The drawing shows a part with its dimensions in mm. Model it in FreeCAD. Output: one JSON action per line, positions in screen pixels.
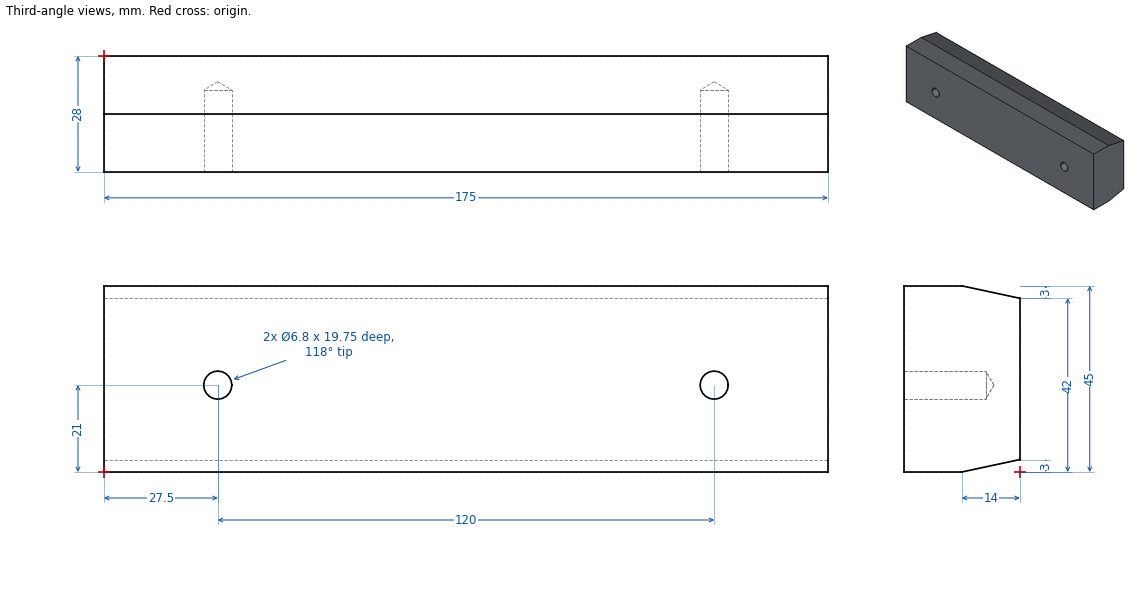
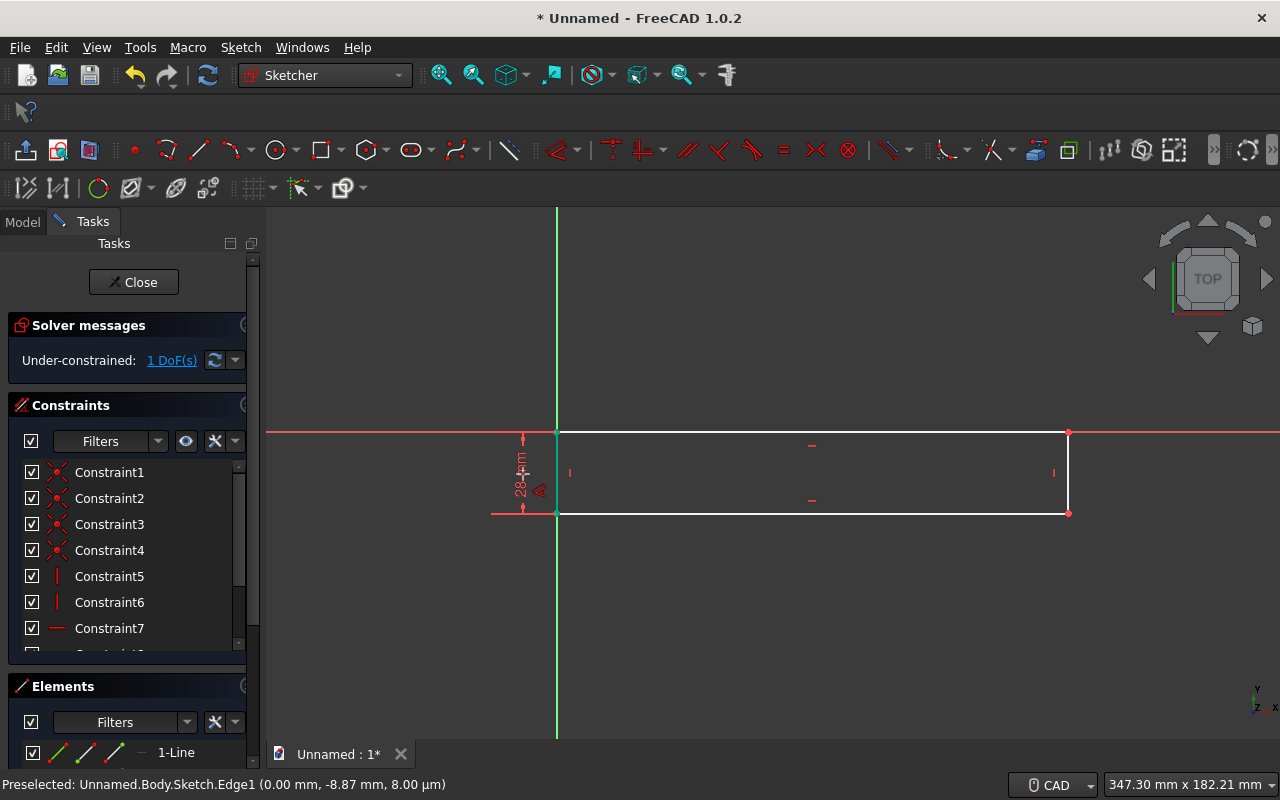
{"action": "left_click", "coordinate": [710, 514]}
{"action": "left_click", "coordinate": [812, 548]}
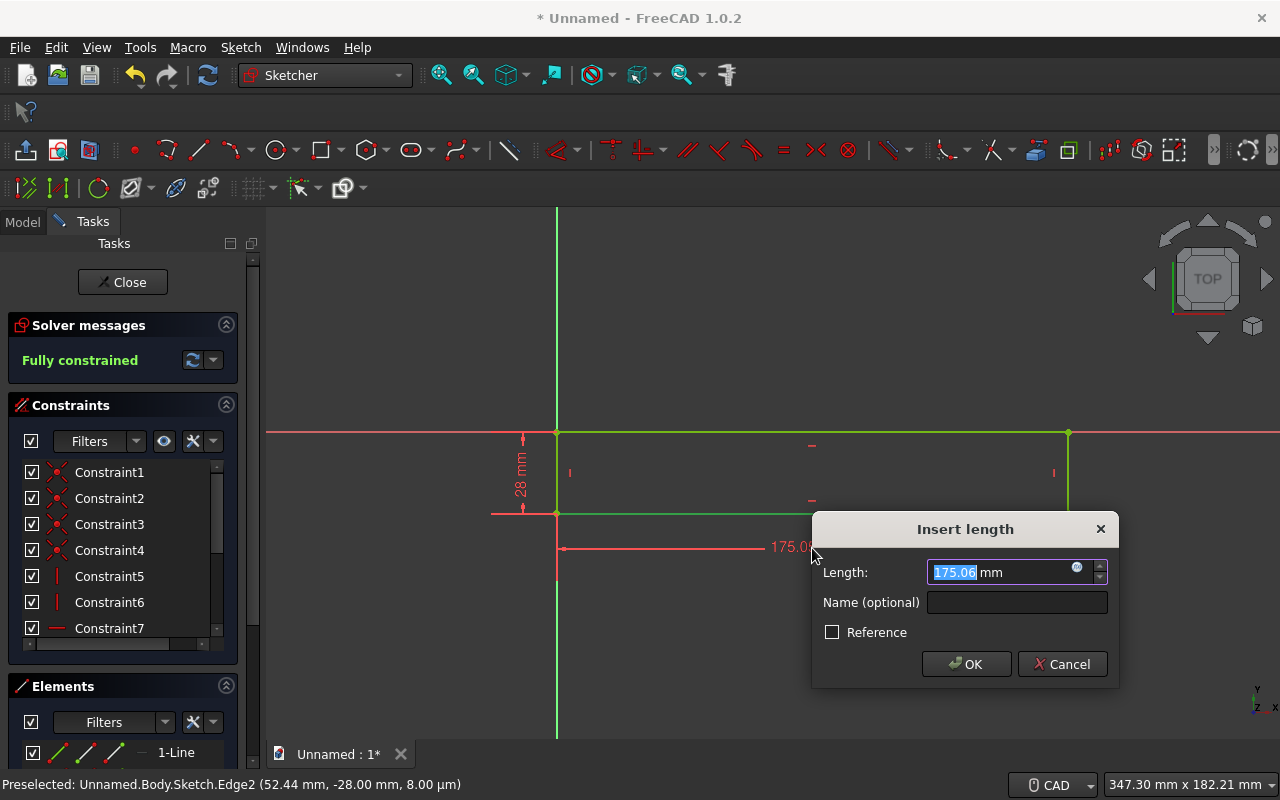
{"action": "type", "text": "175"}
{"action": "key", "text": "Return"}
{"action": "key", "text": "Escape"}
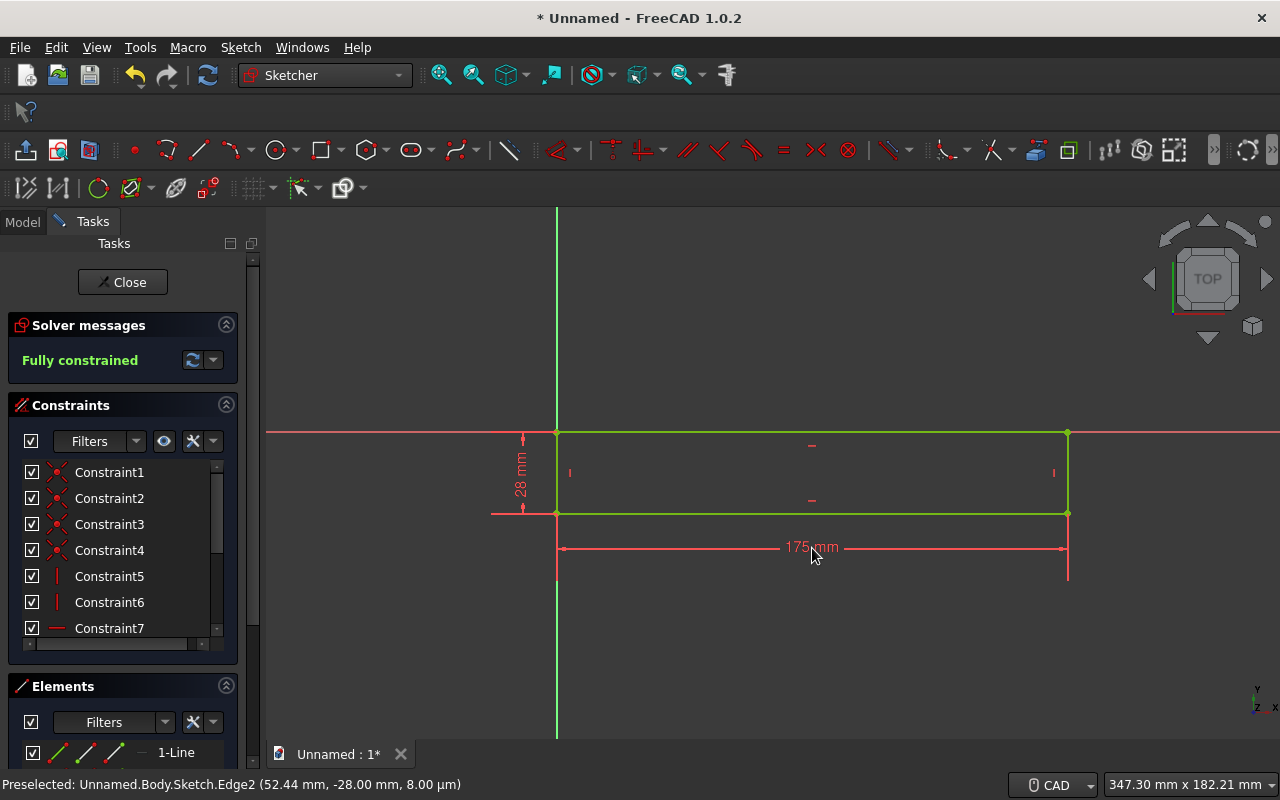
{"action": "left_click", "coordinate": [123, 282]}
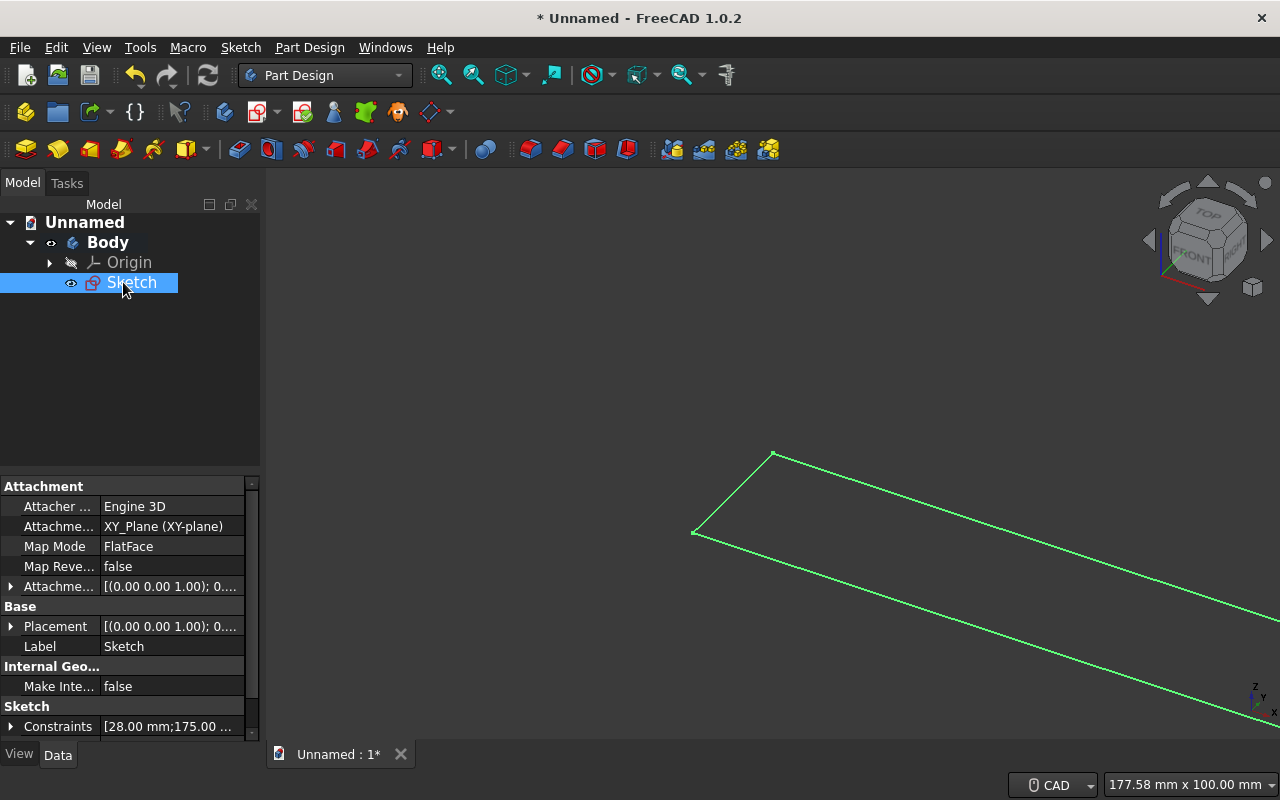
{"action": "left_click", "coordinate": [26, 150]}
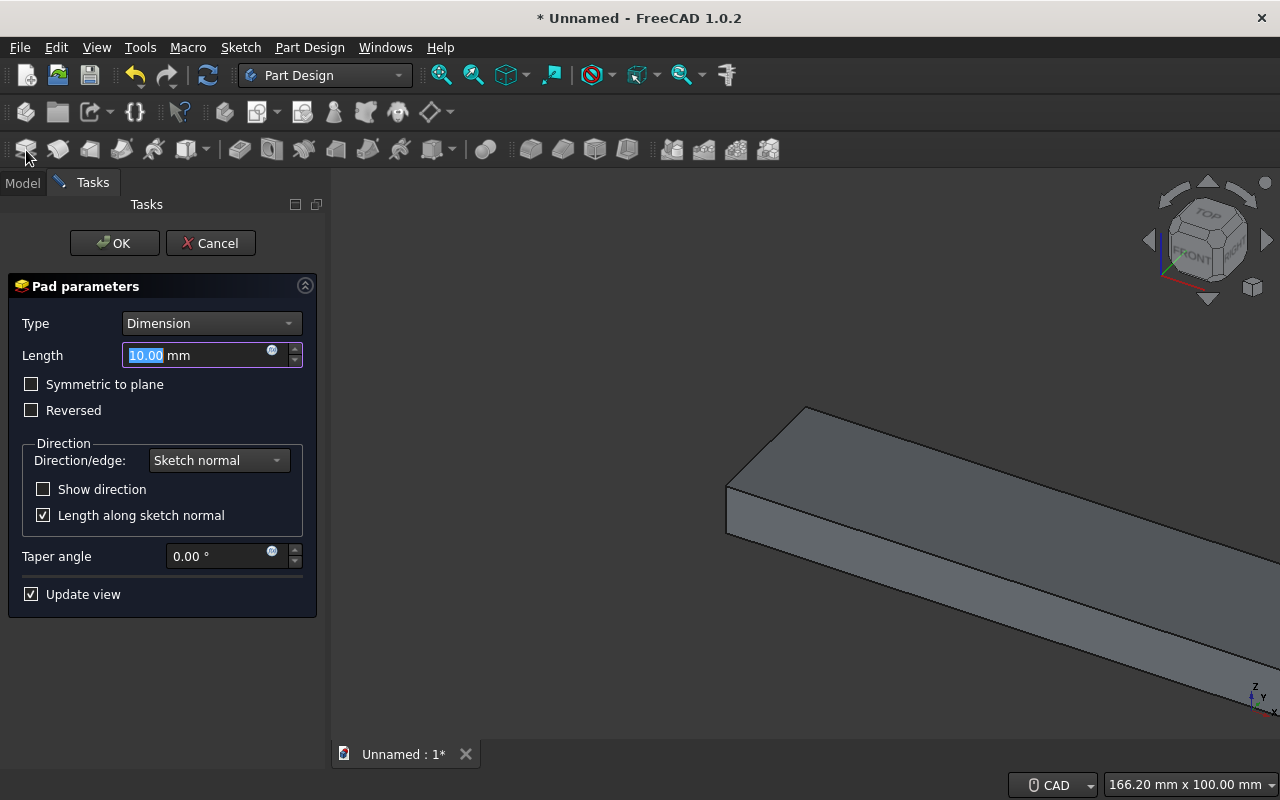
{"action": "type", "text": "45"}
{"action": "key", "text": "Tab"}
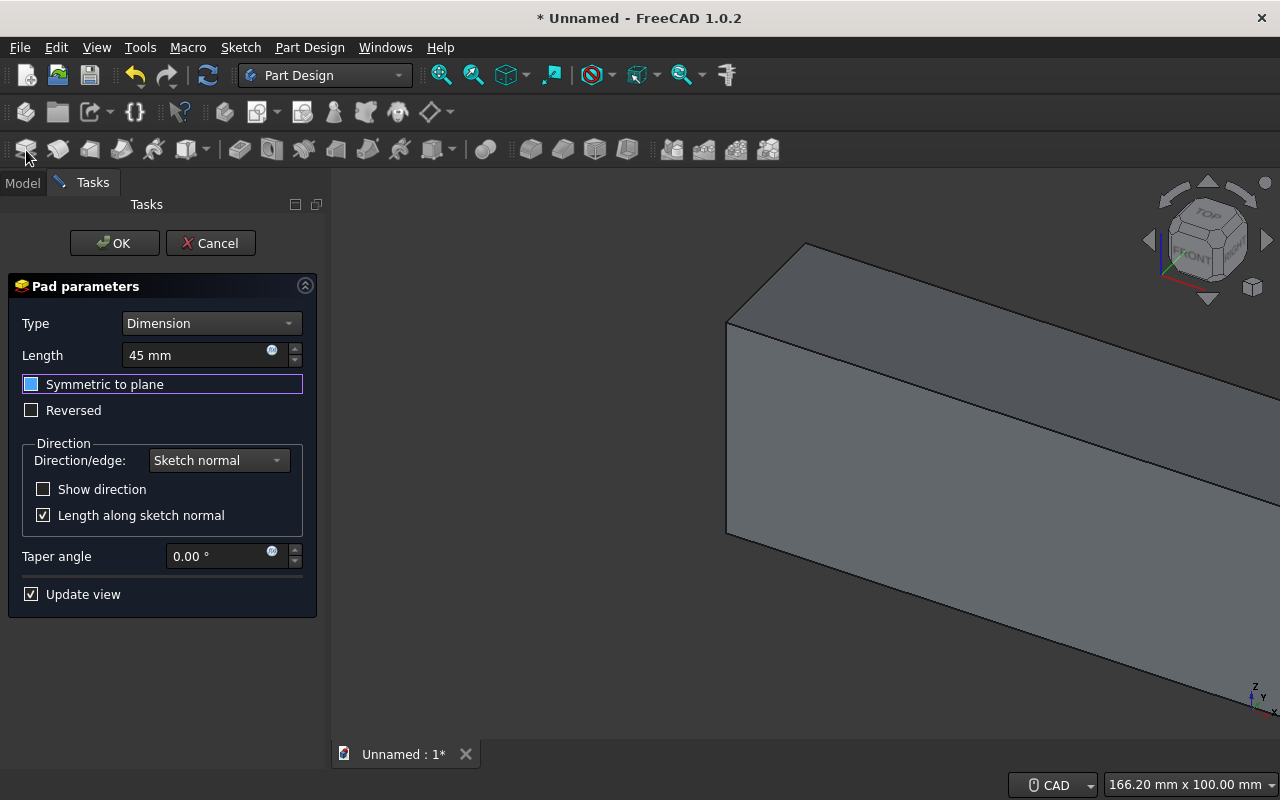
{"action": "left_click", "coordinate": [115, 243]}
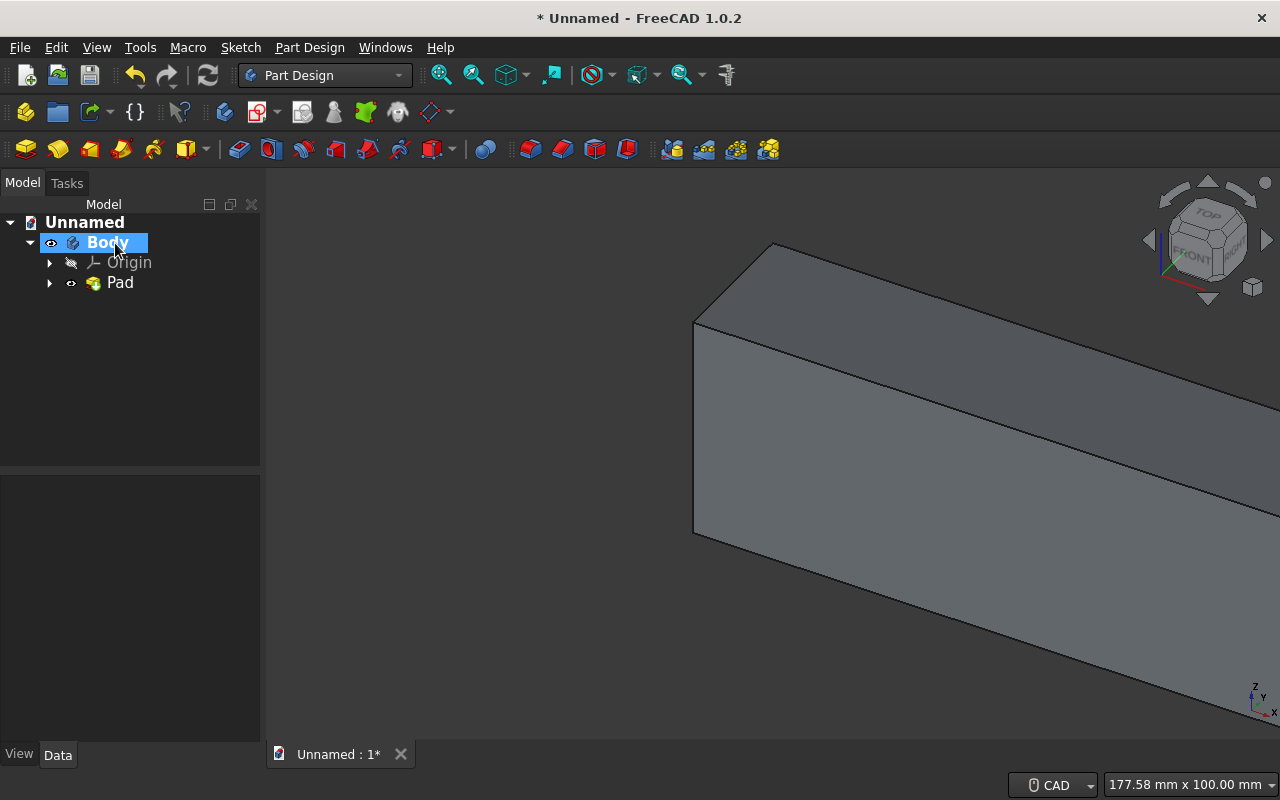
{"action": "key", "text": "v f"}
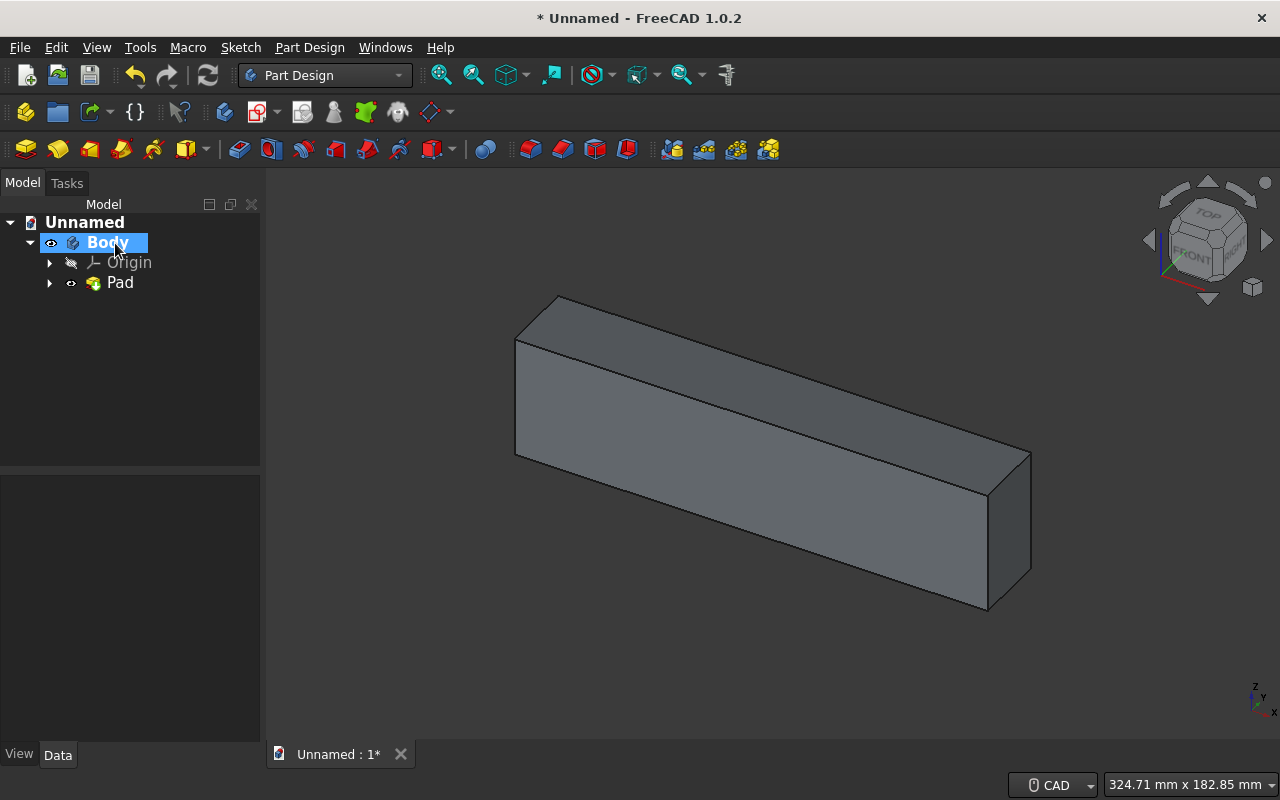
{"action": "left_click", "coordinate": [886, 519]}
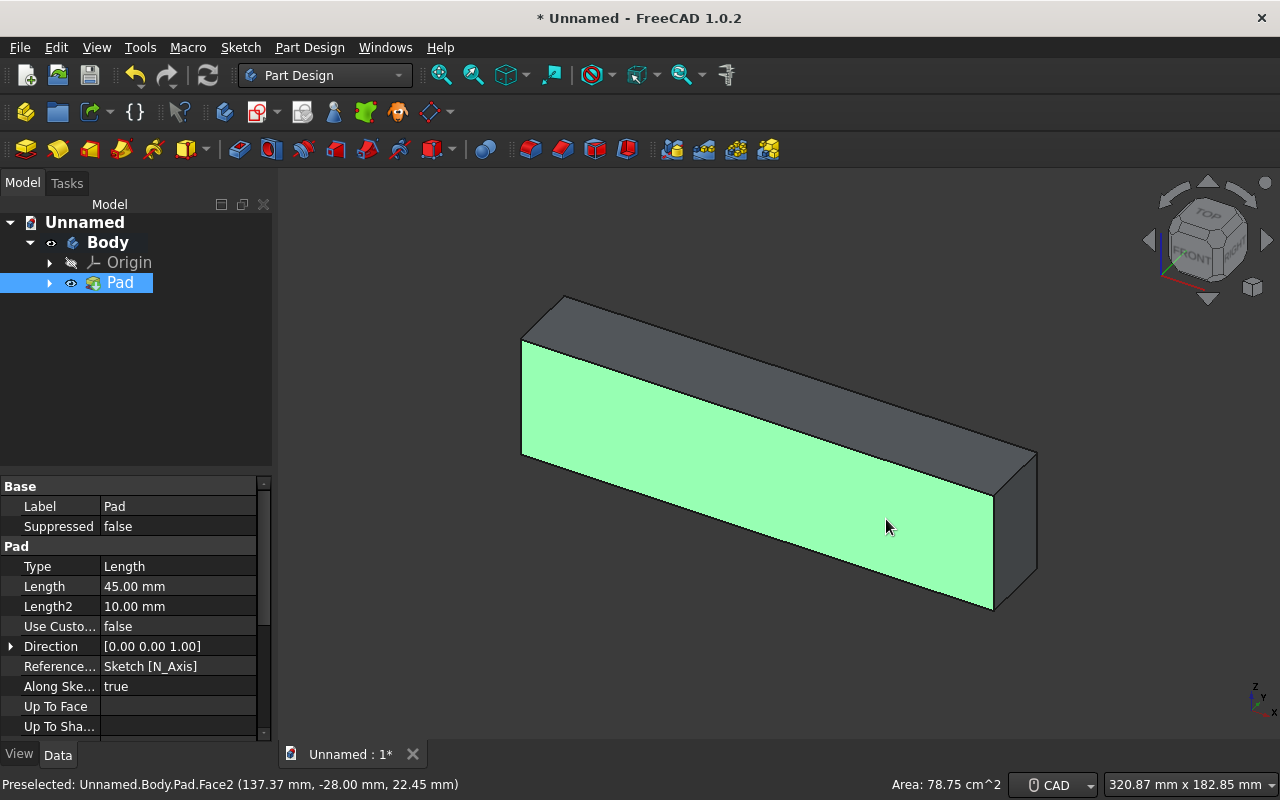
{"action": "left_click", "coordinate": [258, 112]}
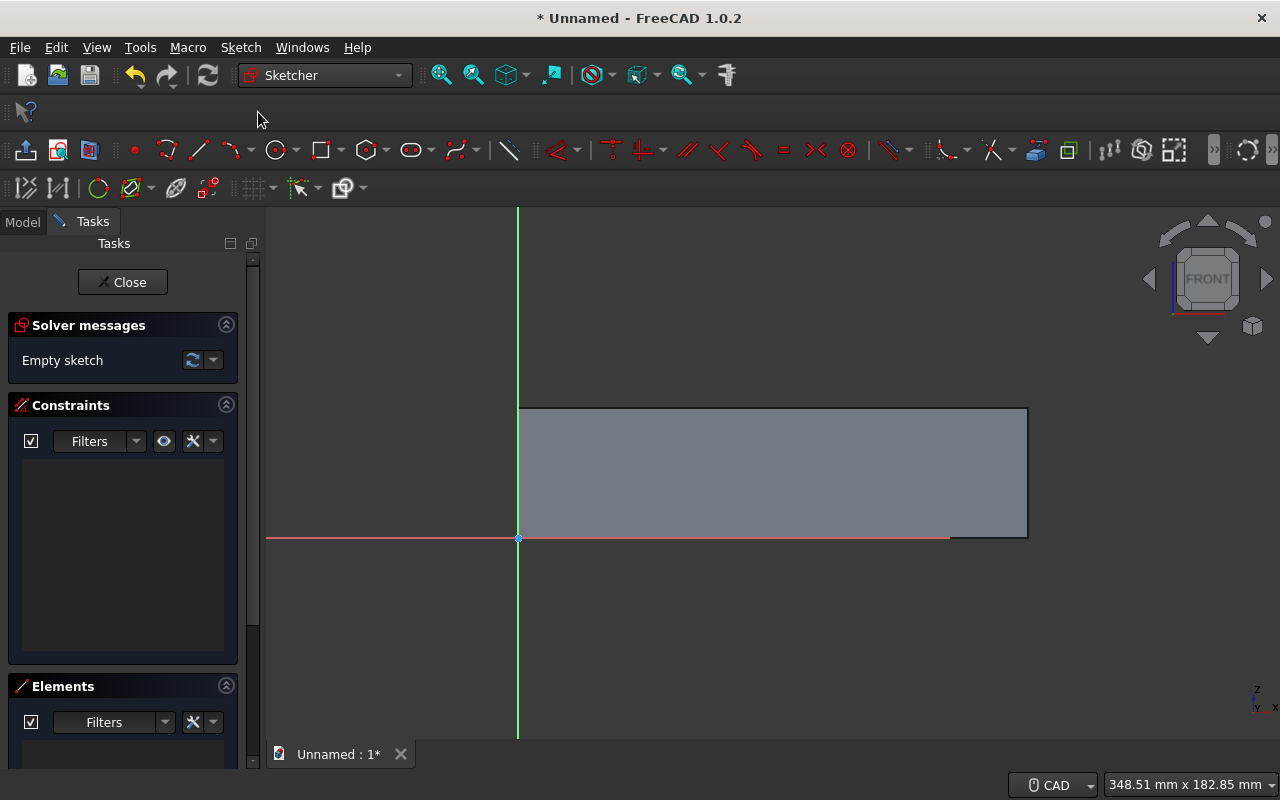
{"action": "left_click", "coordinate": [276, 150]}